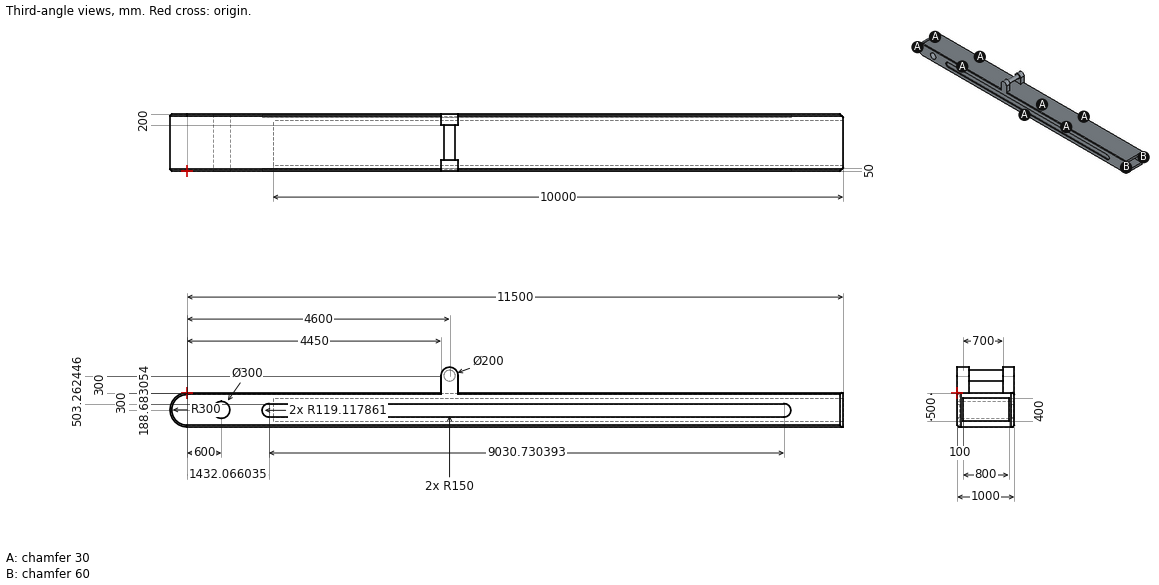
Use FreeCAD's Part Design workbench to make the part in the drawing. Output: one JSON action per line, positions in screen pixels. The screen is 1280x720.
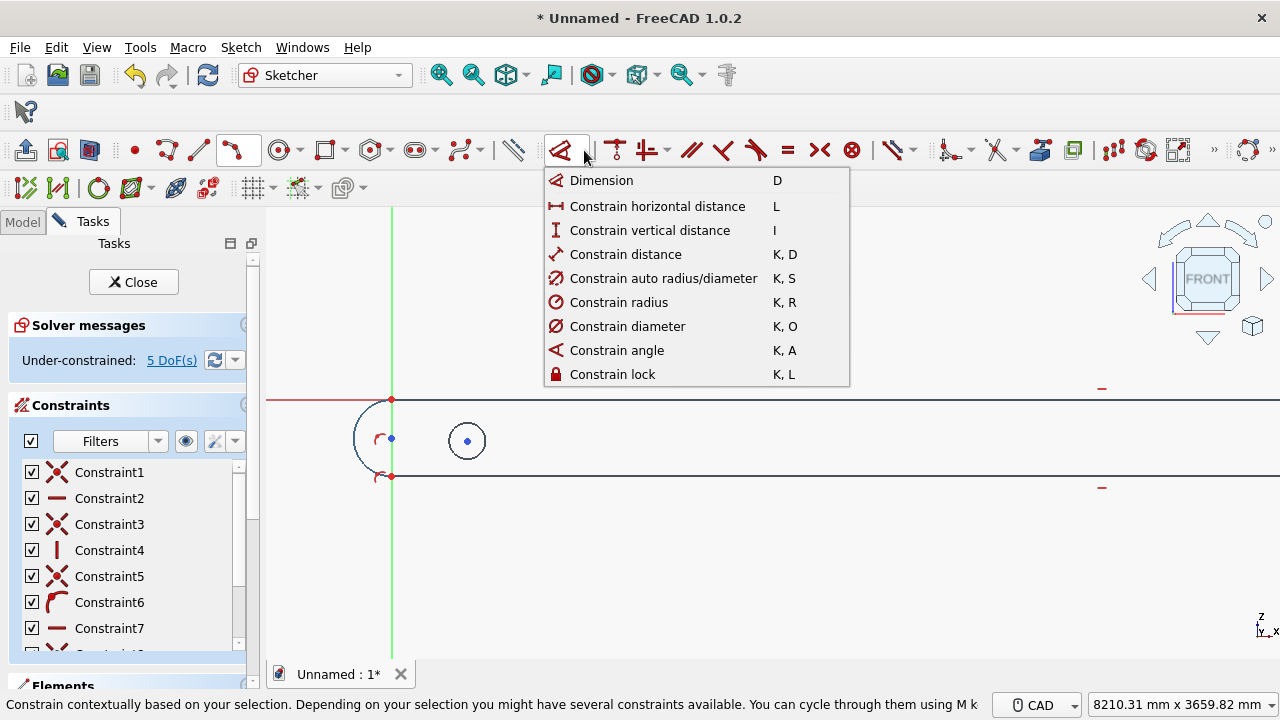
{"action": "left_click", "coordinate": [697, 302]}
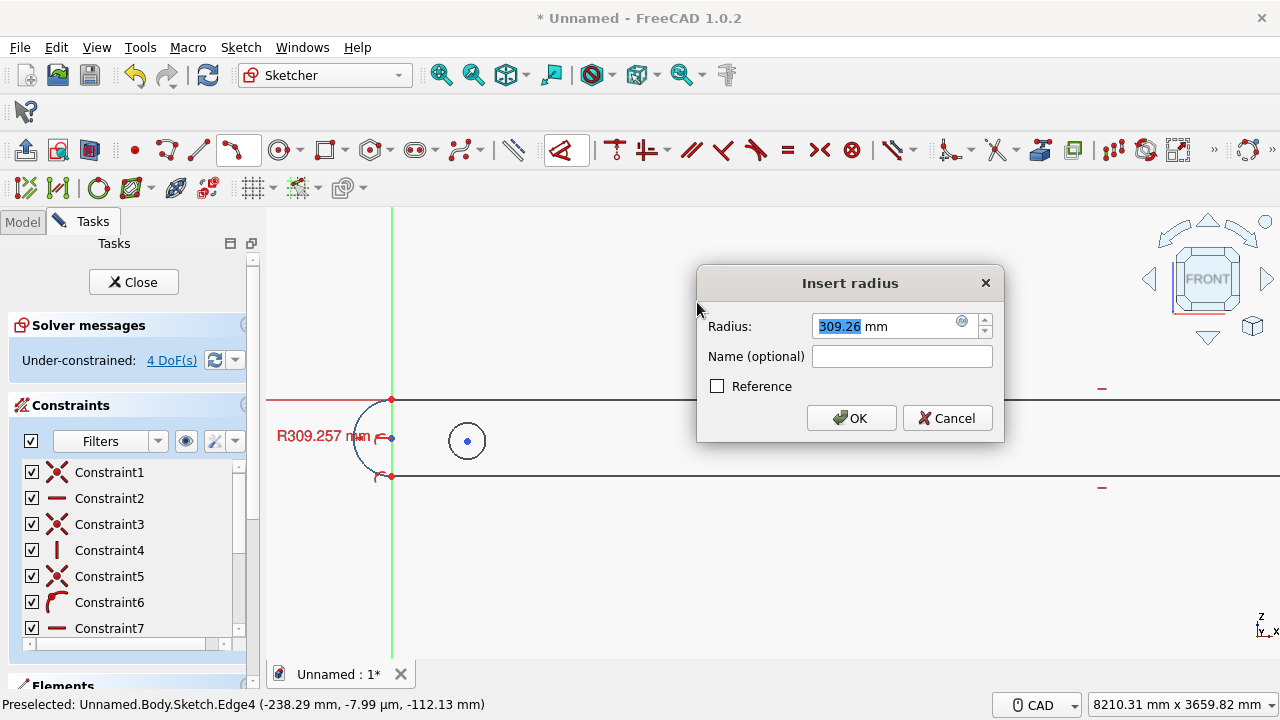
{"action": "type", "text": "300"}
{"action": "key", "text": "Return"}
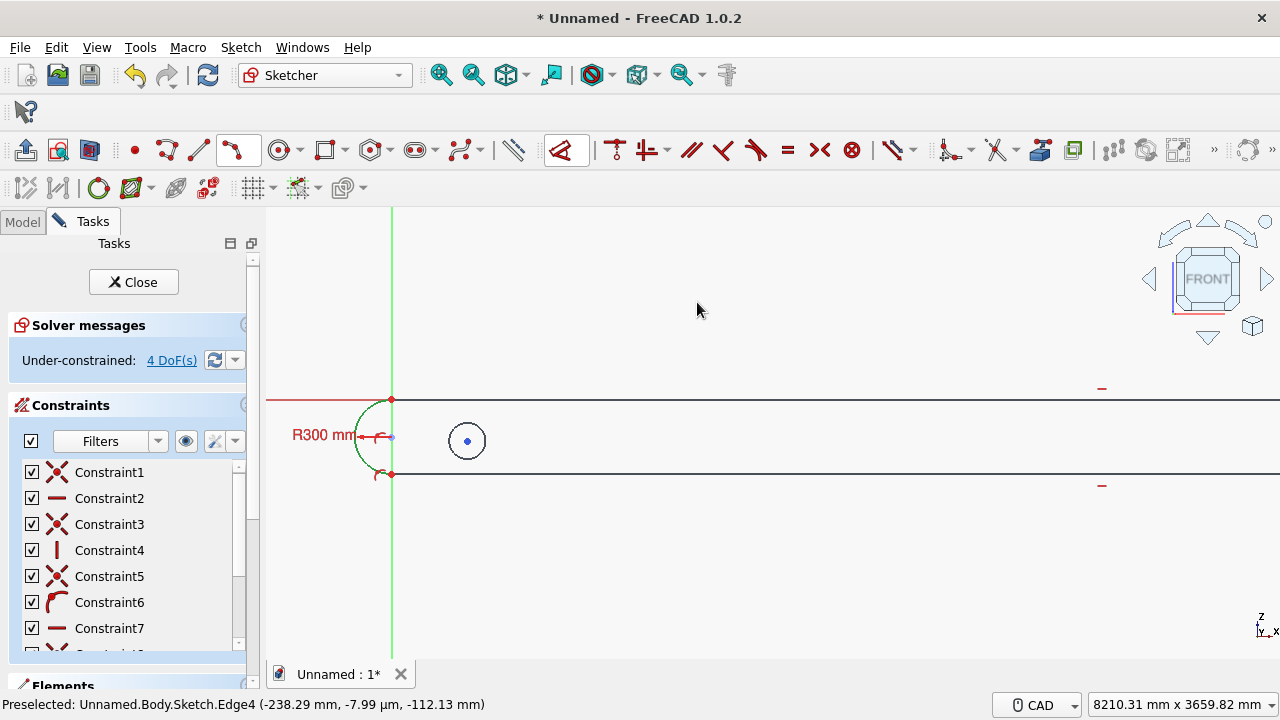
{"action": "left_click", "coordinate": [480, 428]}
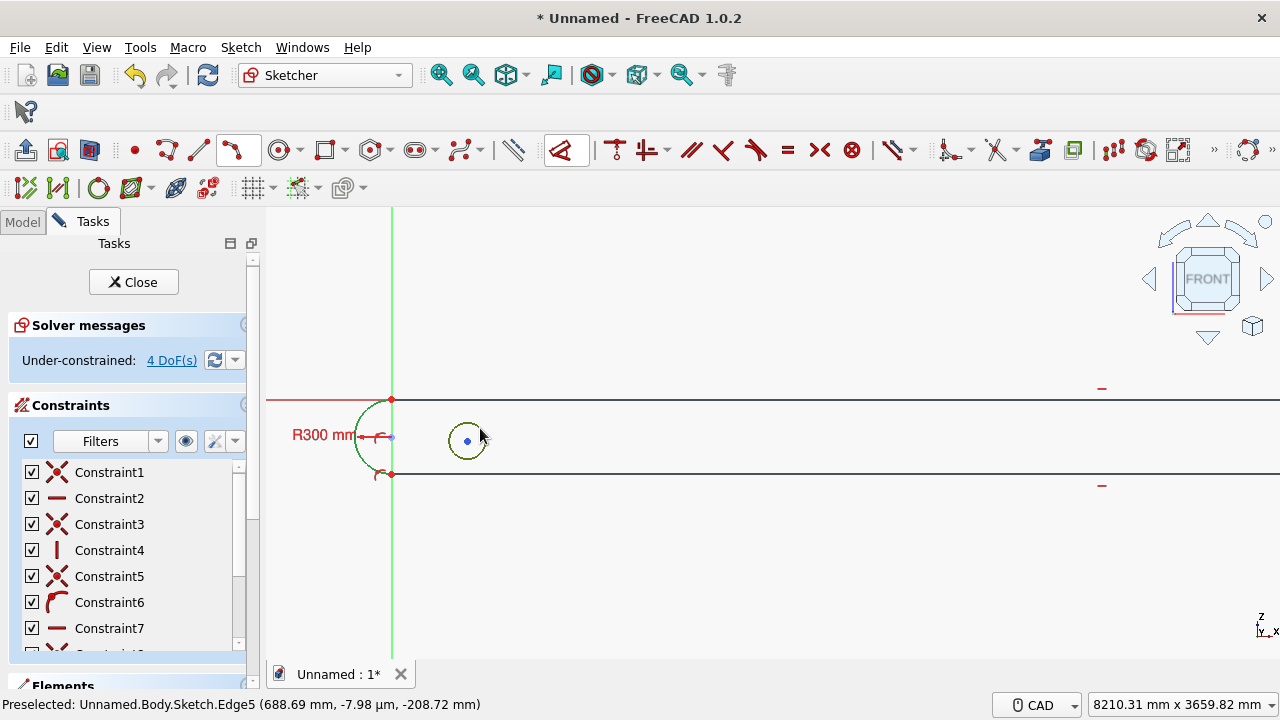
{"action": "left_click", "coordinate": [584, 150]}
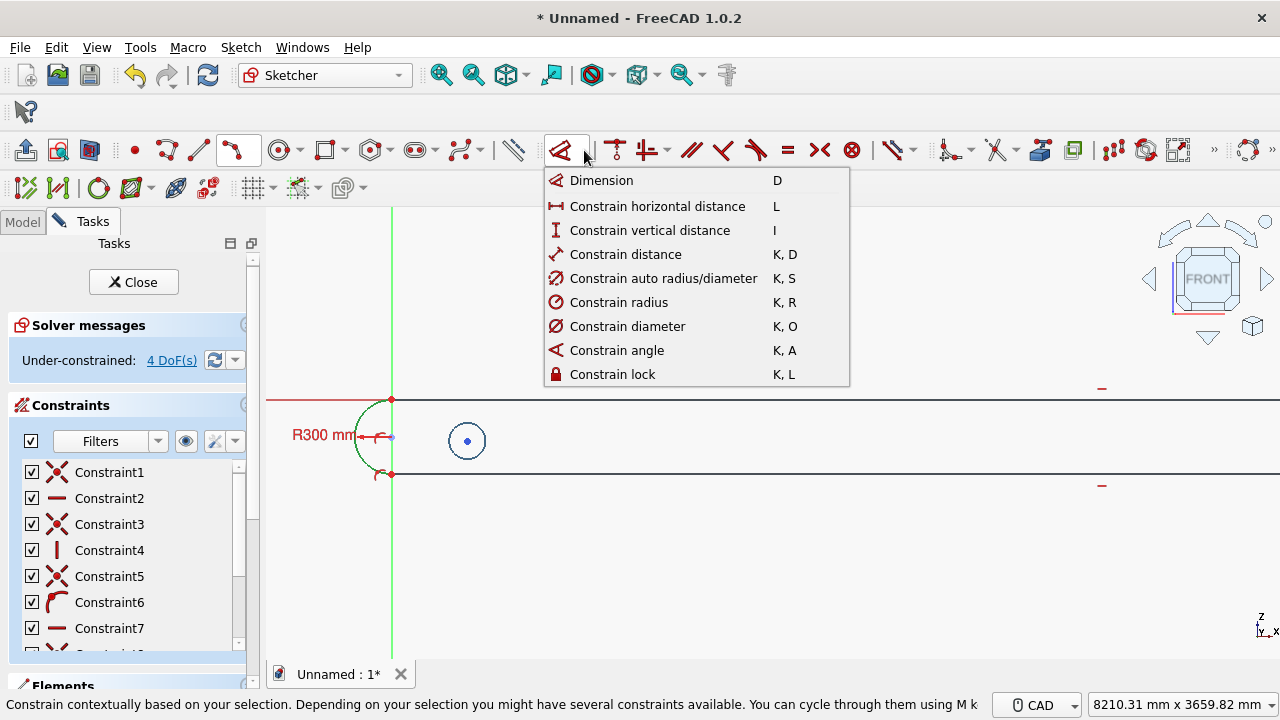
{"action": "left_click", "coordinate": [697, 326]}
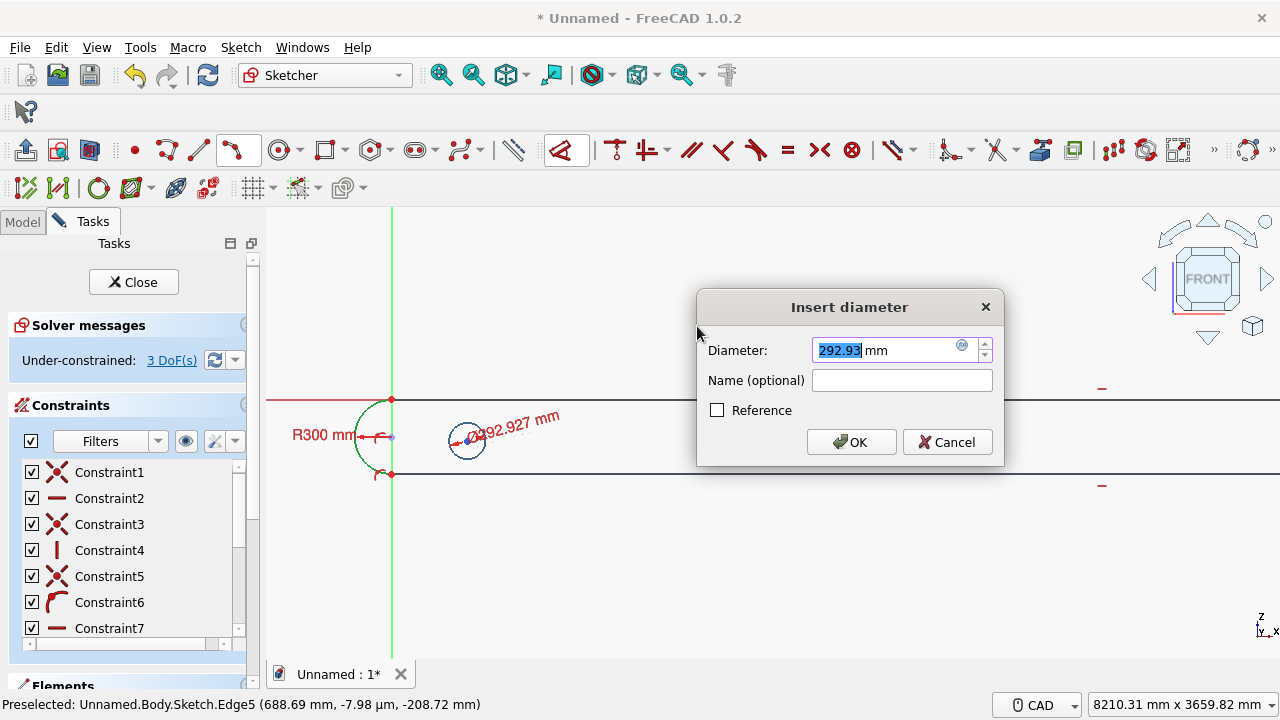
{"action": "type", "text": "300"}
{"action": "key", "text": "Return"}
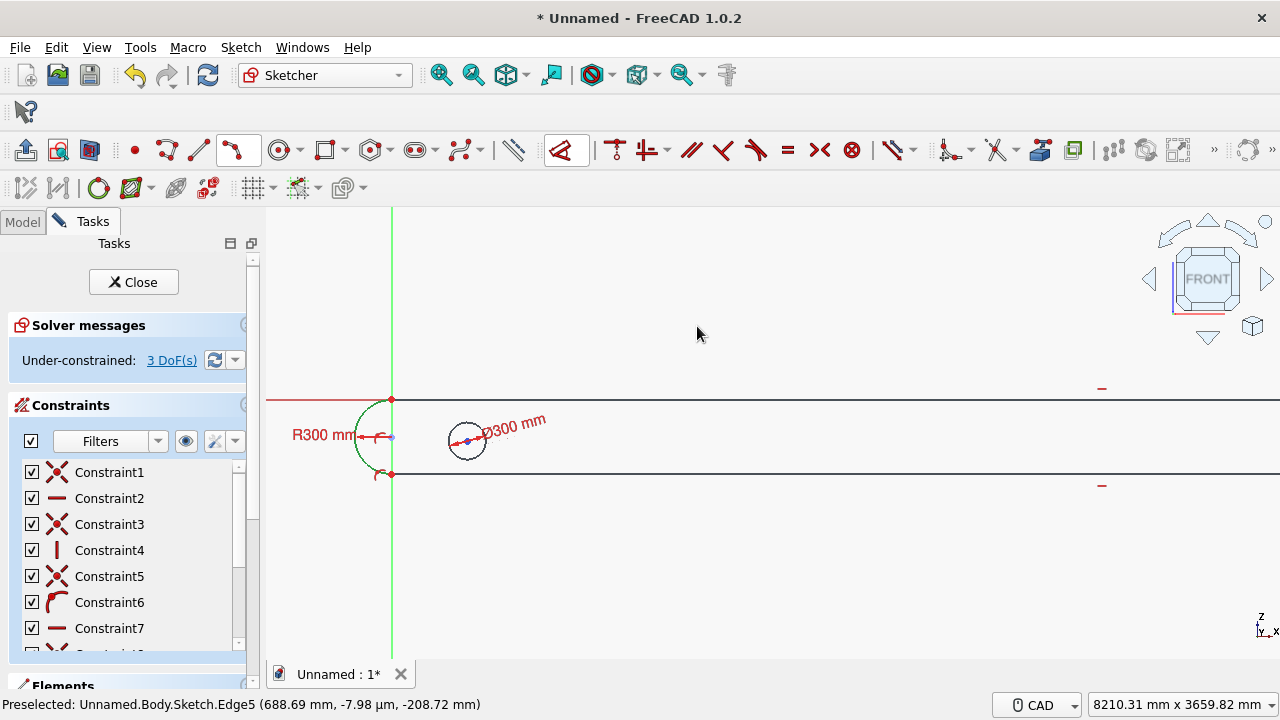
{"action": "left_click", "coordinate": [467, 441]}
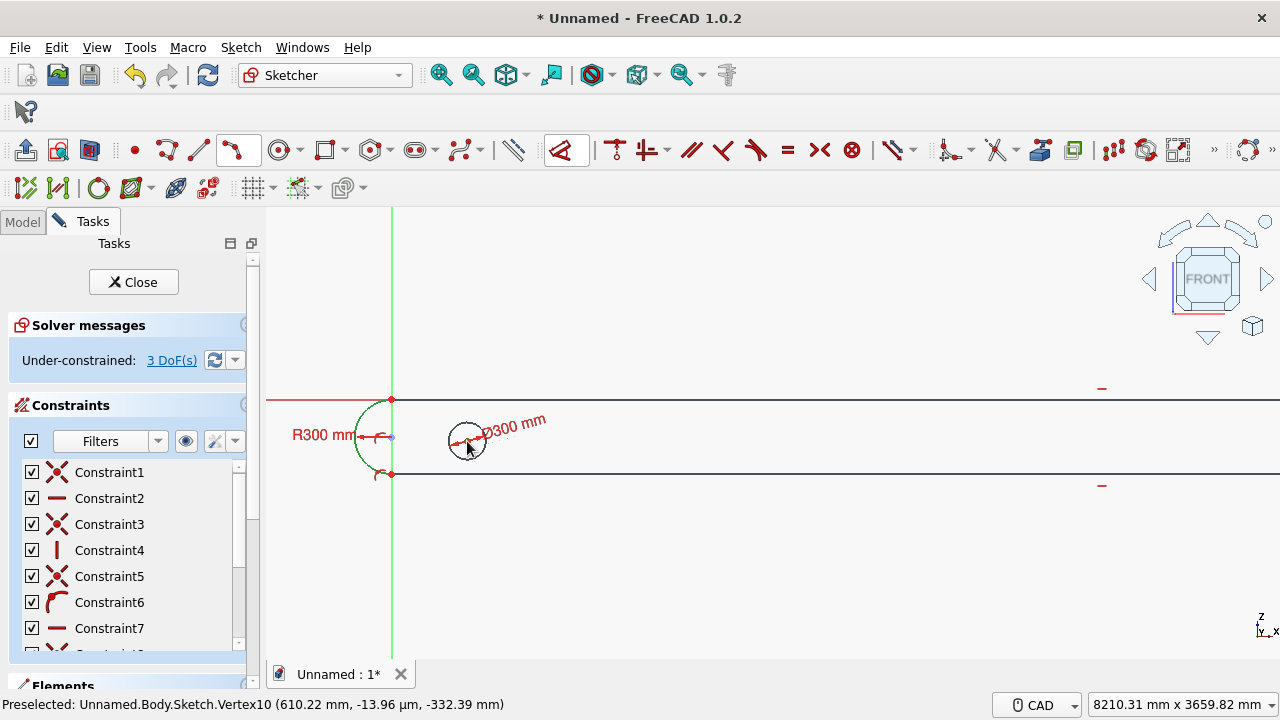
{"action": "left_click", "coordinate": [584, 150]}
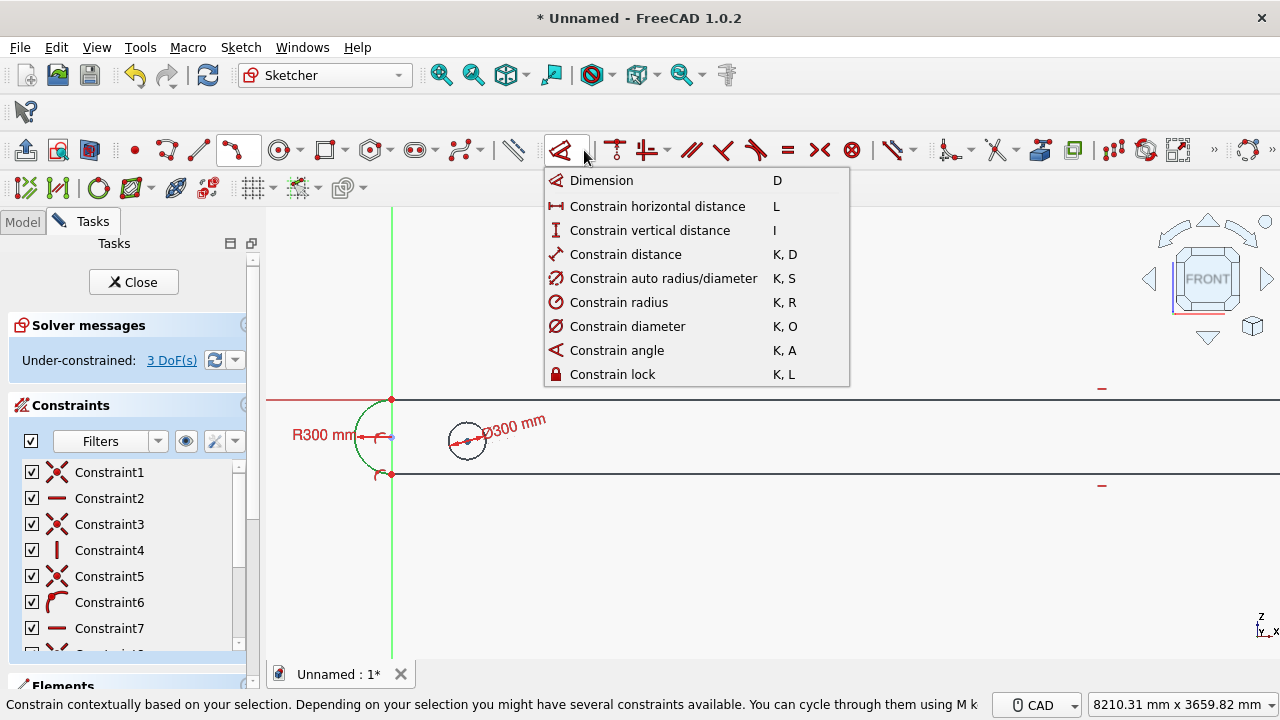
{"action": "left_click", "coordinate": [697, 206]}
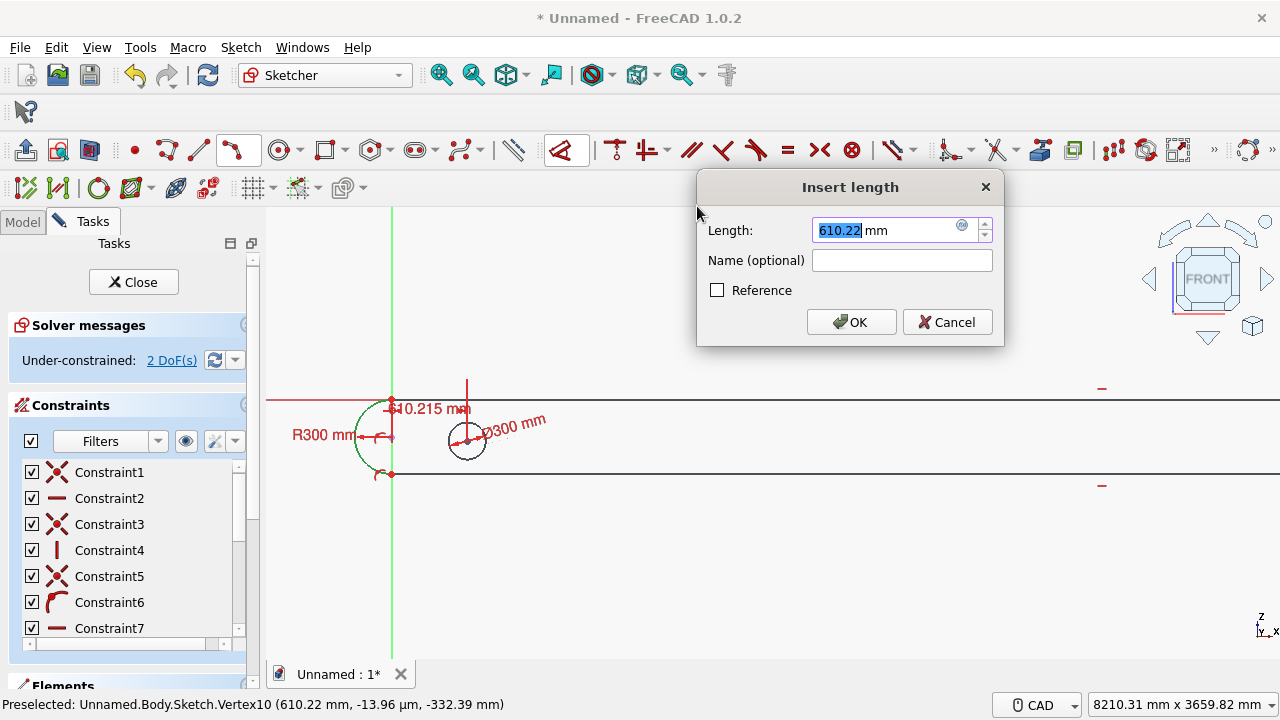
{"action": "type", "text": "600"}
{"action": "key", "text": "Return"}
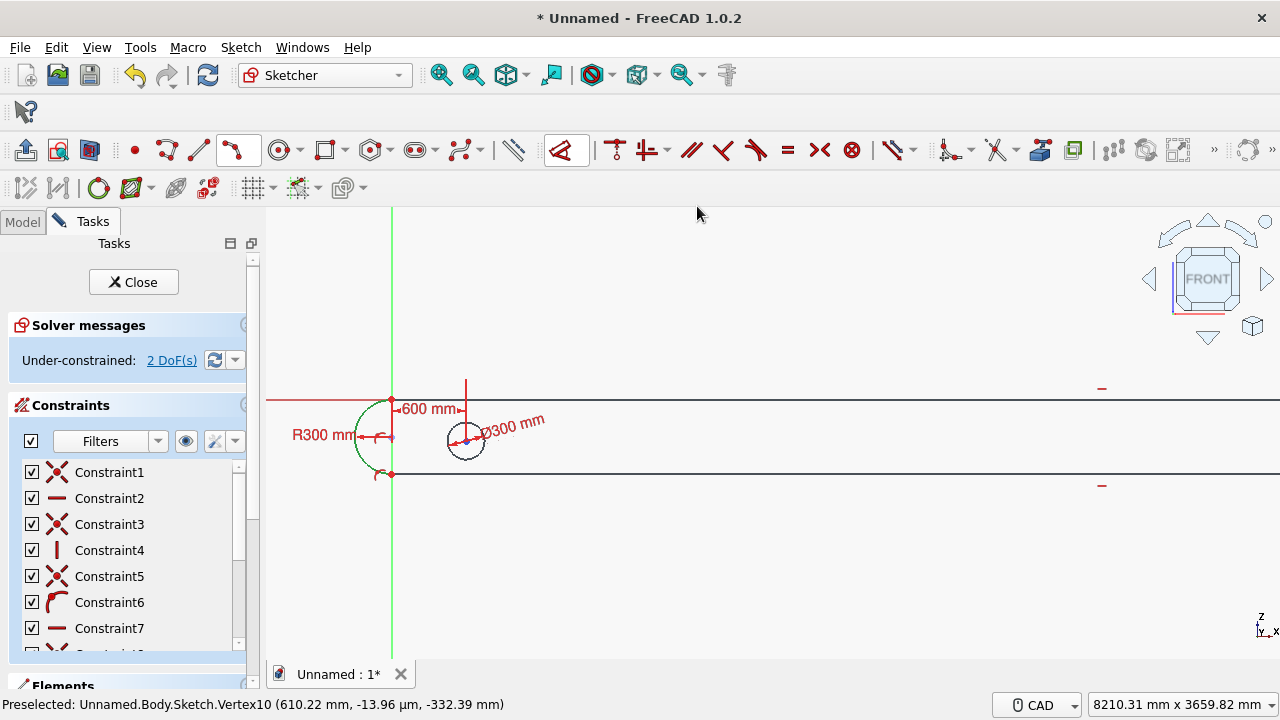
{"action": "left_click", "coordinate": [466, 441]}